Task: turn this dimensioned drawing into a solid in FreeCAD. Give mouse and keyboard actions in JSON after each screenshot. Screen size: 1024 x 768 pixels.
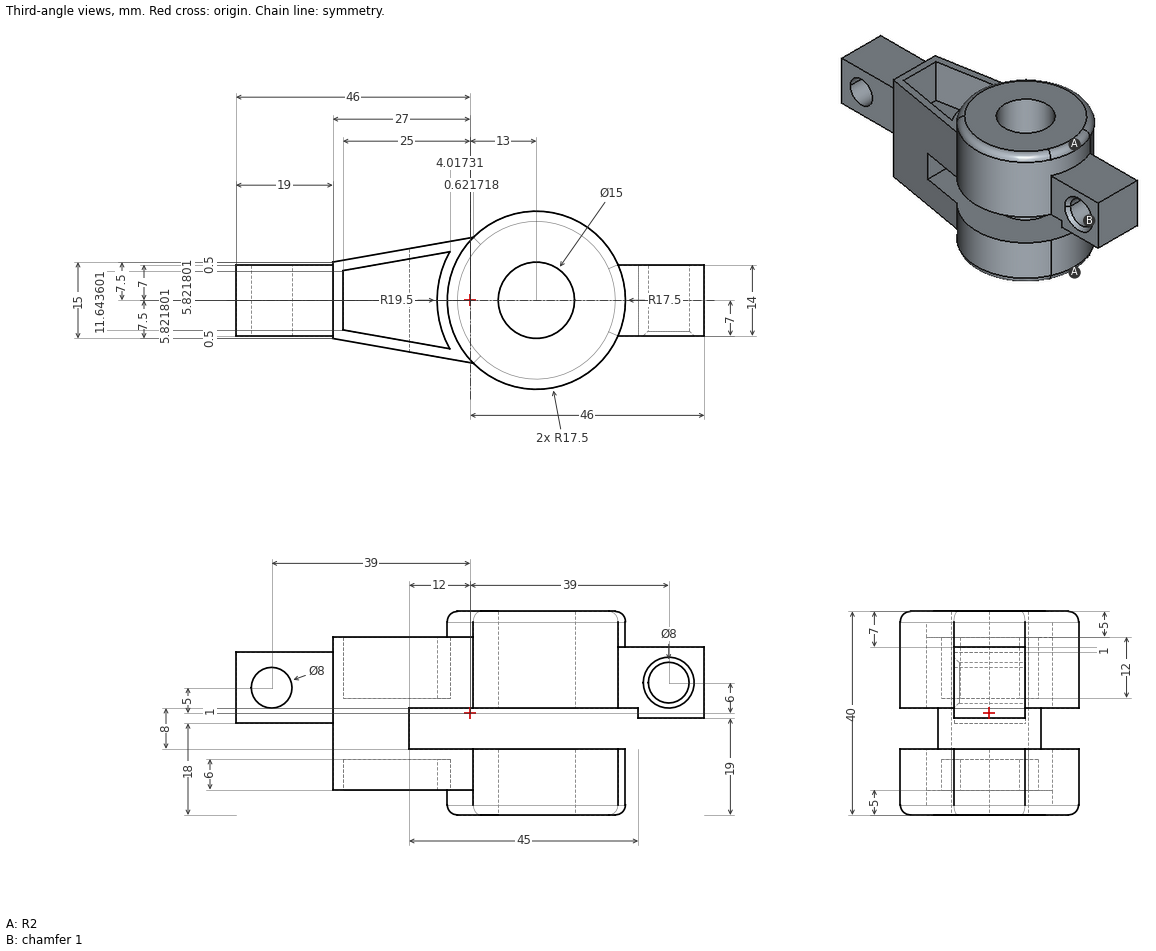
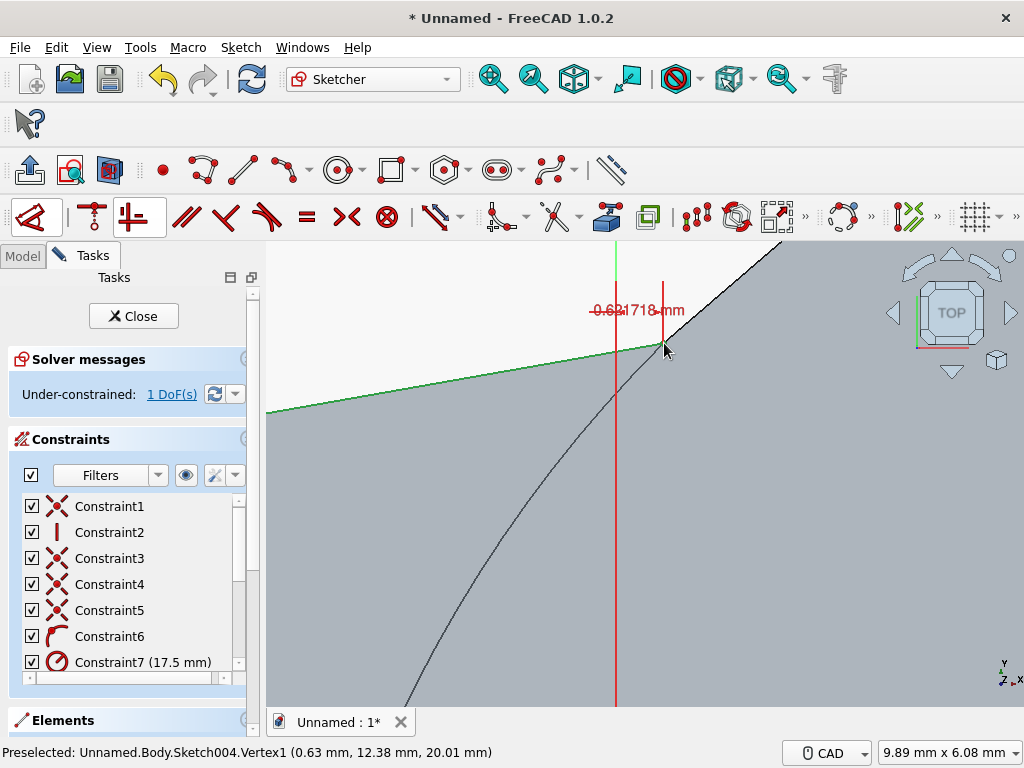
{"action": "scroll", "coordinate": [769, 312], "scroll_direction": "down", "scroll_amount": 9}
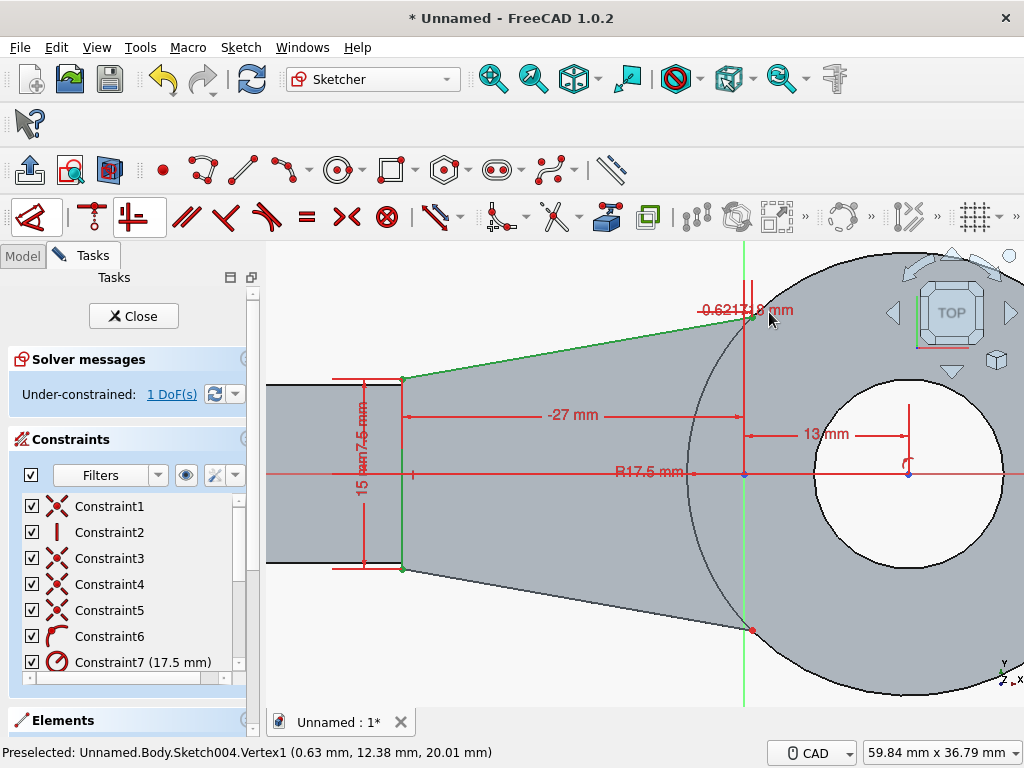
{"action": "scroll", "coordinate": [752, 631], "scroll_direction": "up", "scroll_amount": 9}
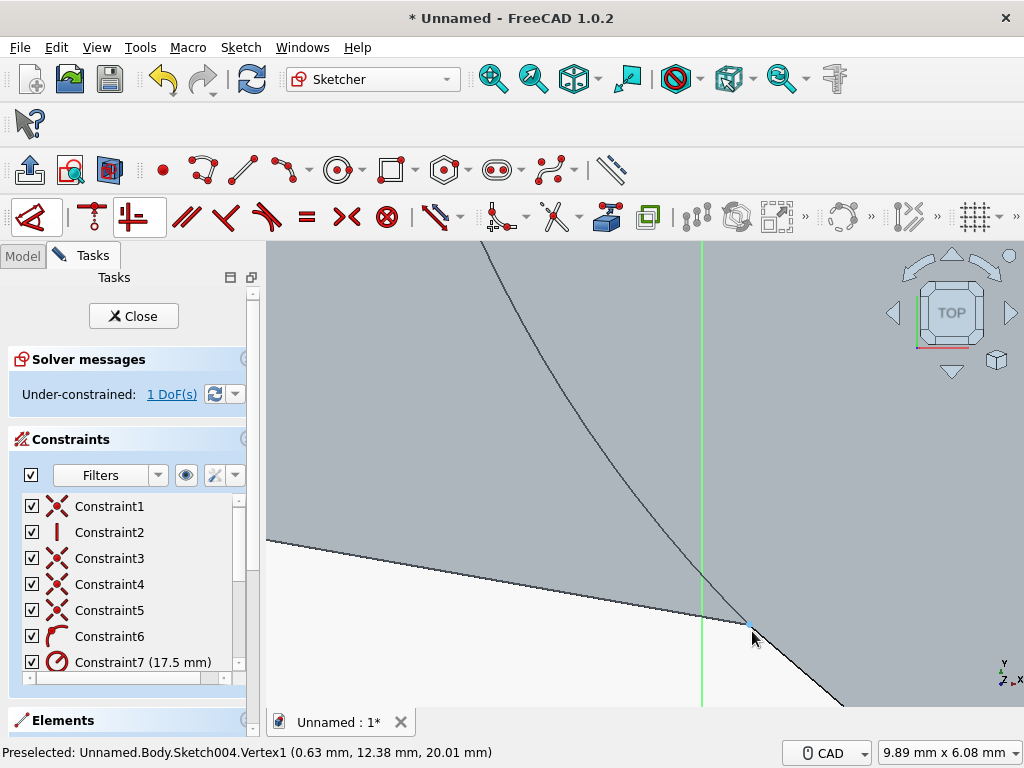
{"action": "left_click", "coordinate": [749, 625]}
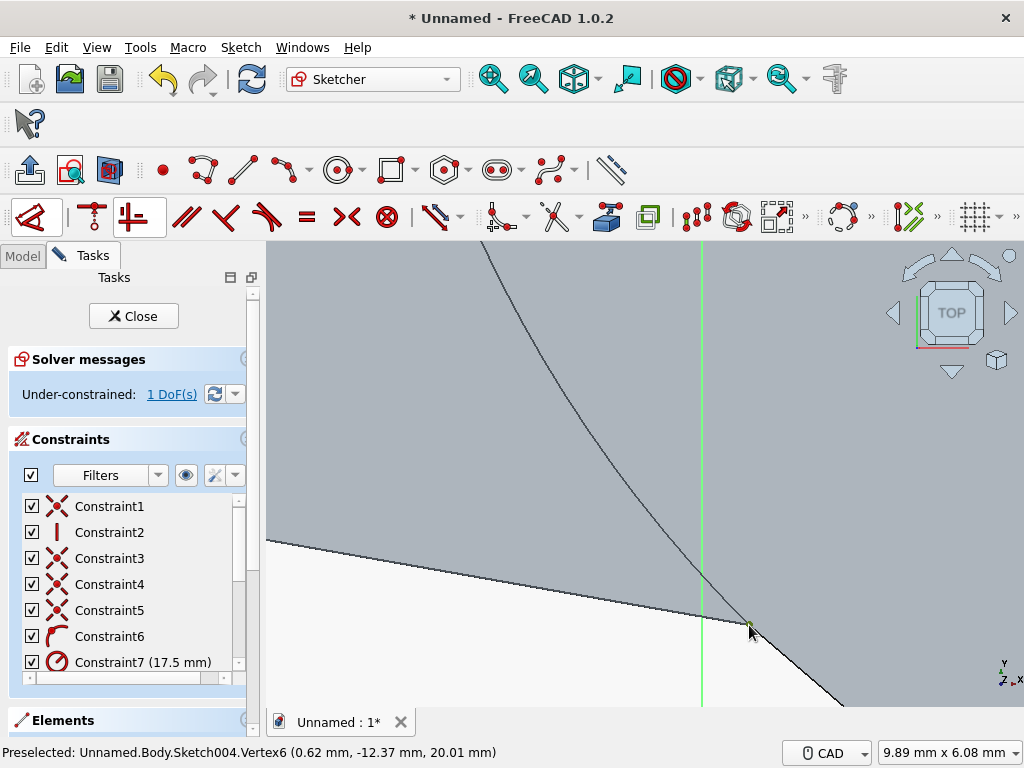
{"action": "key", "text": "l"}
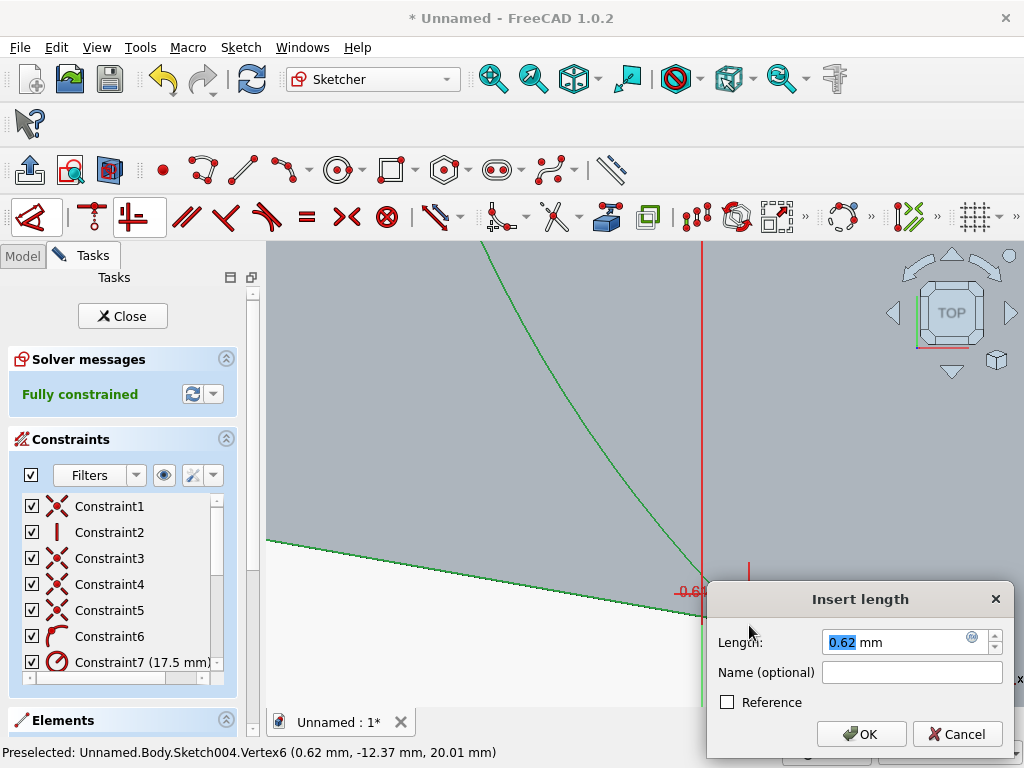
{"action": "type", "text": "0.621718"}
{"action": "key", "text": "Return"}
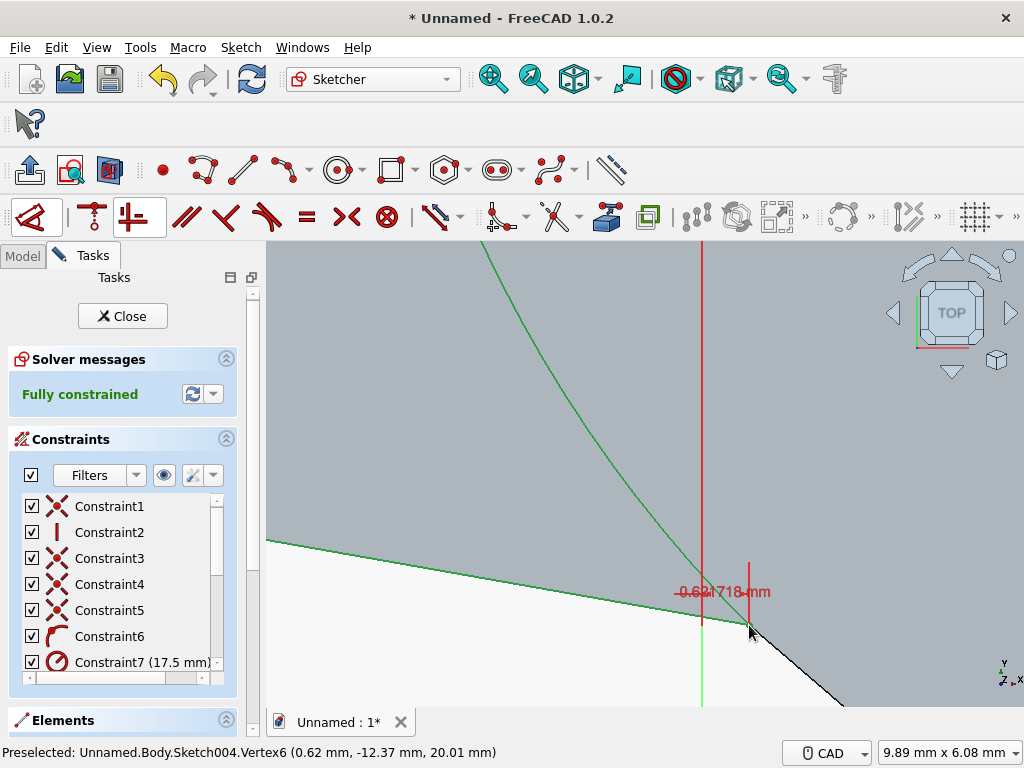
{"action": "left_click", "coordinate": [123, 316]}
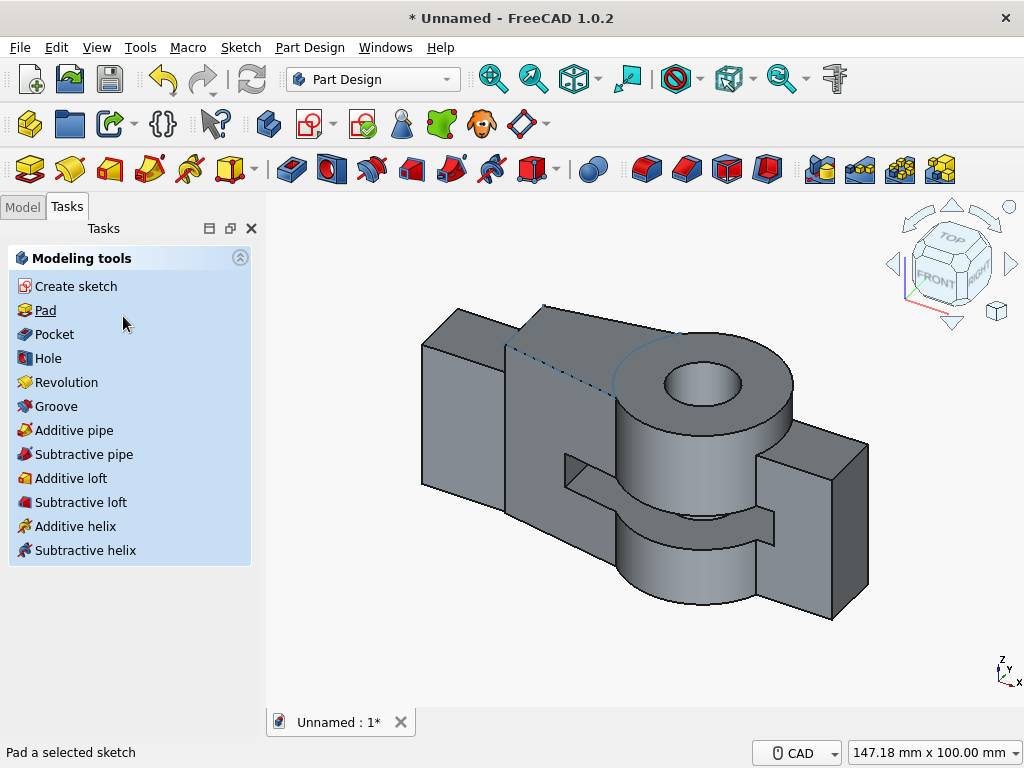
{"action": "left_click", "coordinate": [292, 170]}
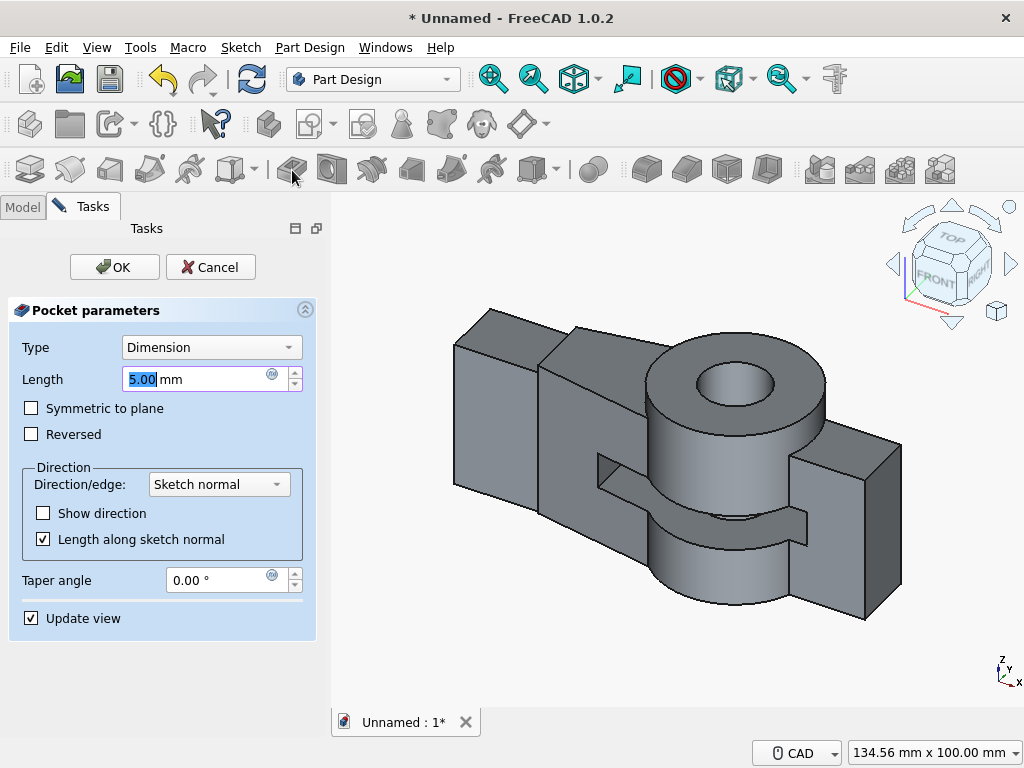
{"action": "type", "text": "5"}
{"action": "key", "text": "Tab"}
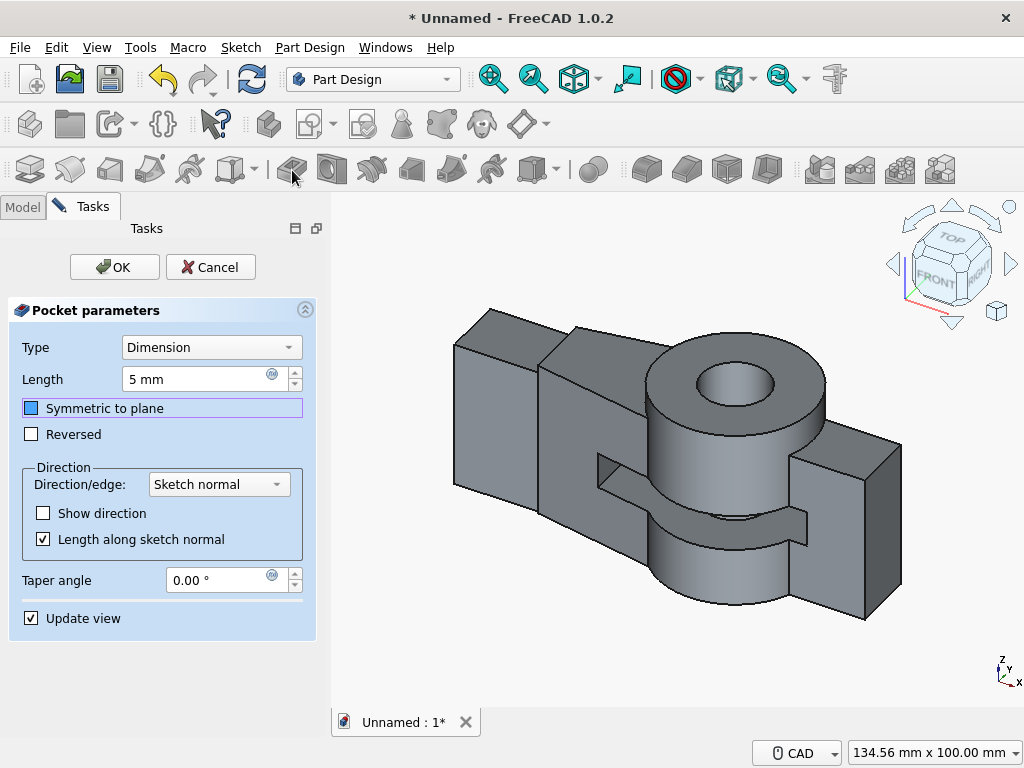
{"action": "left_click", "coordinate": [115, 267]}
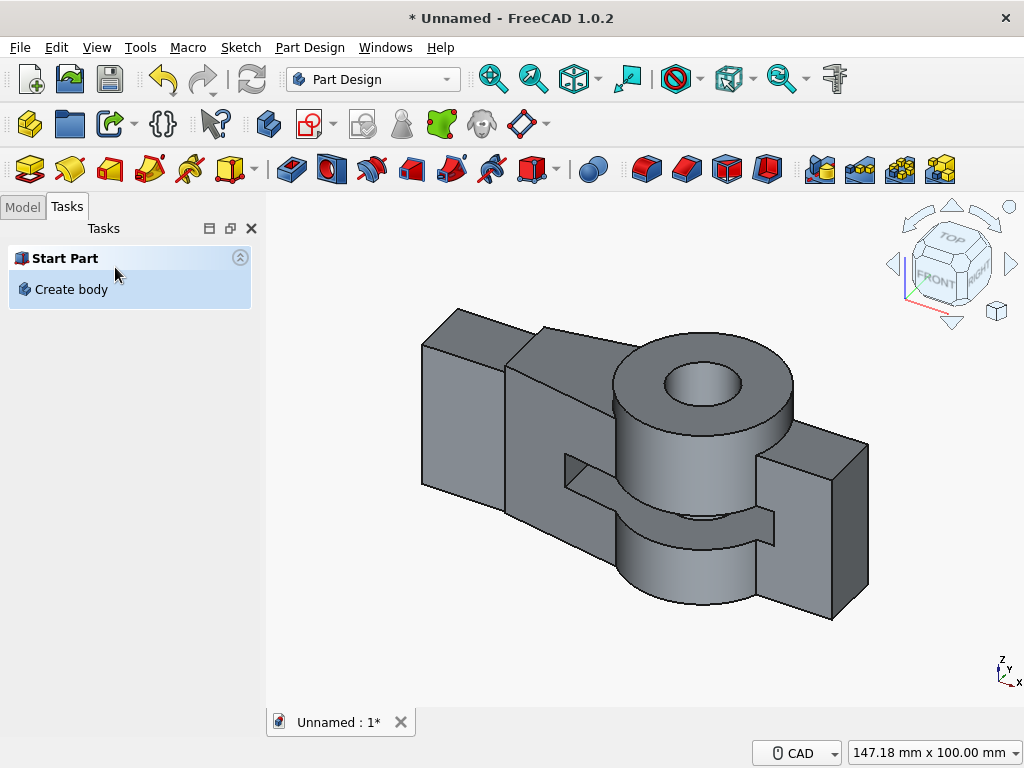
{"action": "left_click", "coordinate": [23, 206]}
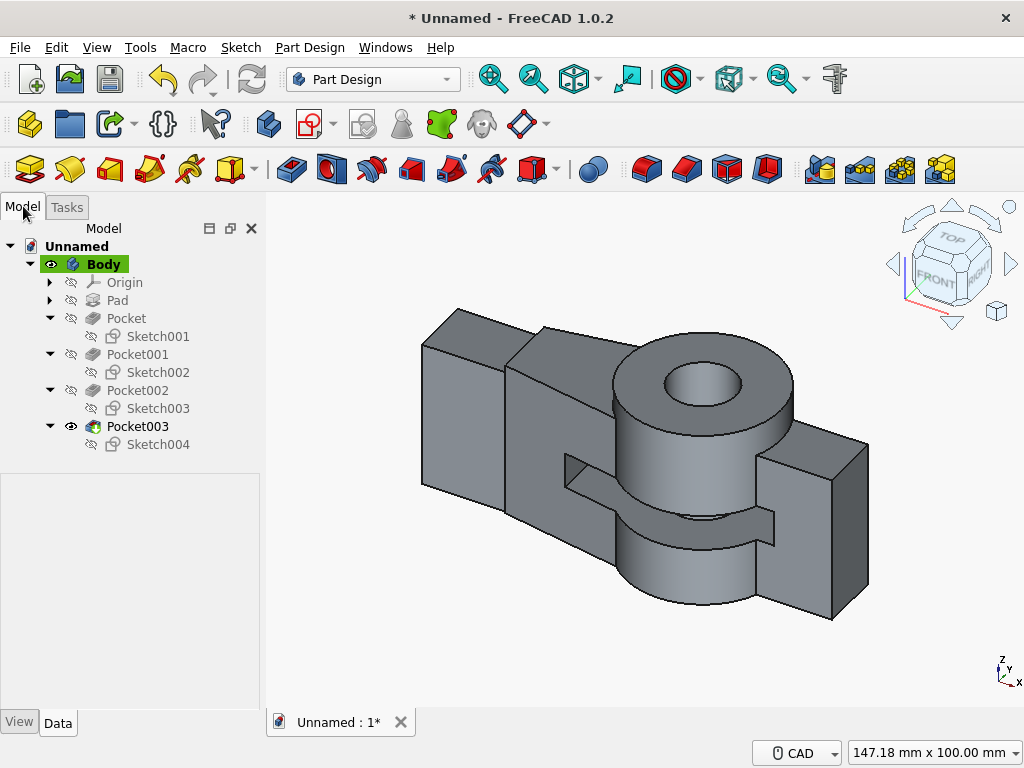
{"action": "left_click", "coordinate": [50, 282]}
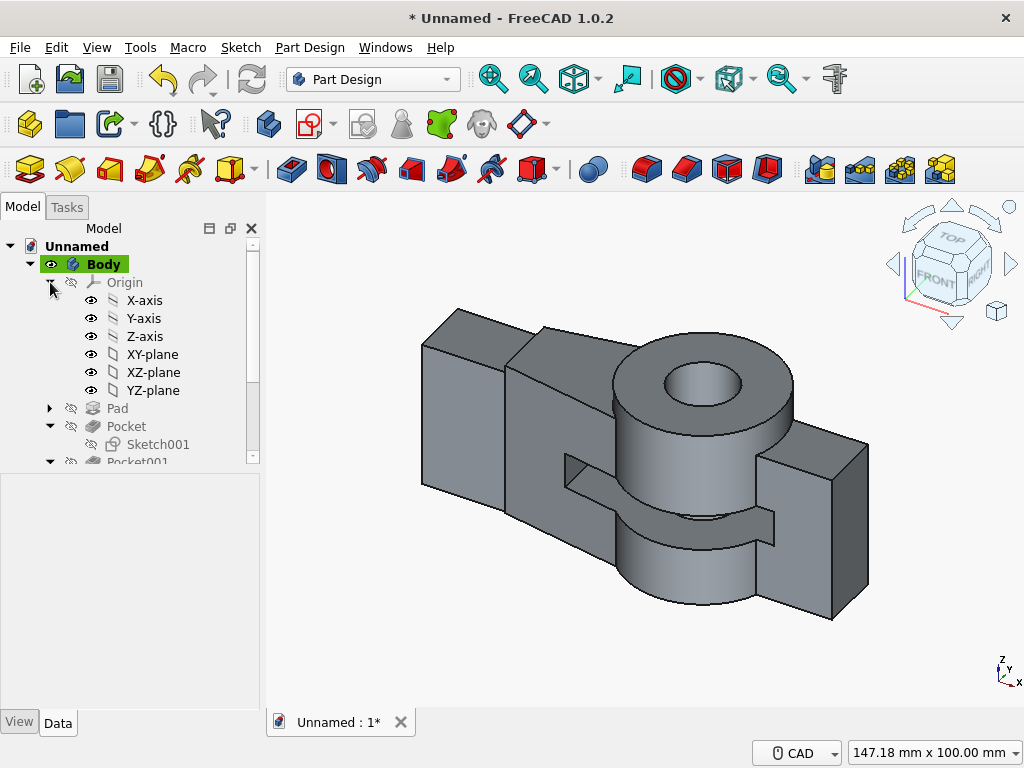
{"action": "left_click", "coordinate": [136, 354]}